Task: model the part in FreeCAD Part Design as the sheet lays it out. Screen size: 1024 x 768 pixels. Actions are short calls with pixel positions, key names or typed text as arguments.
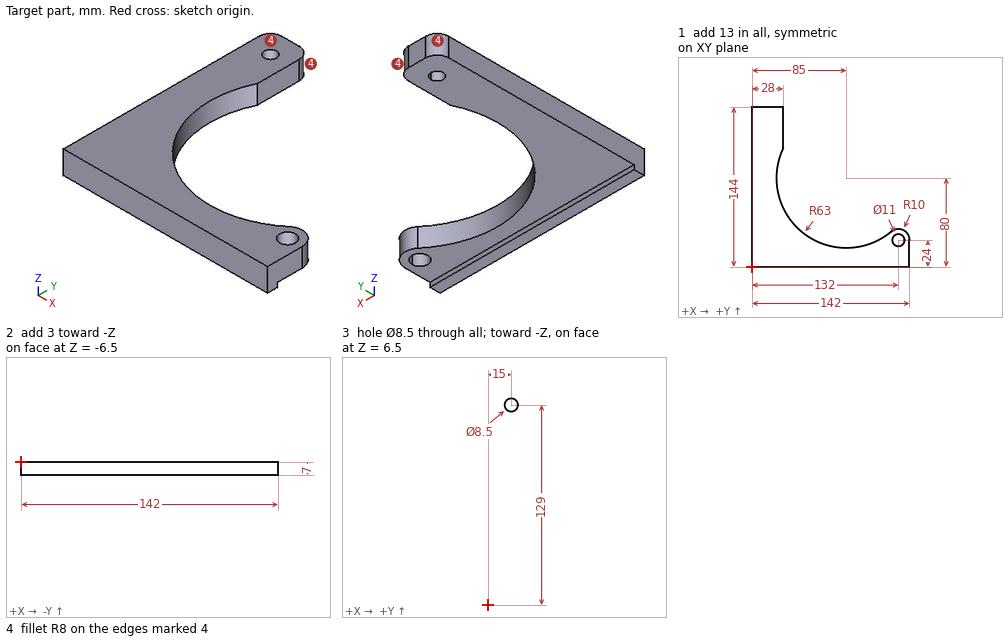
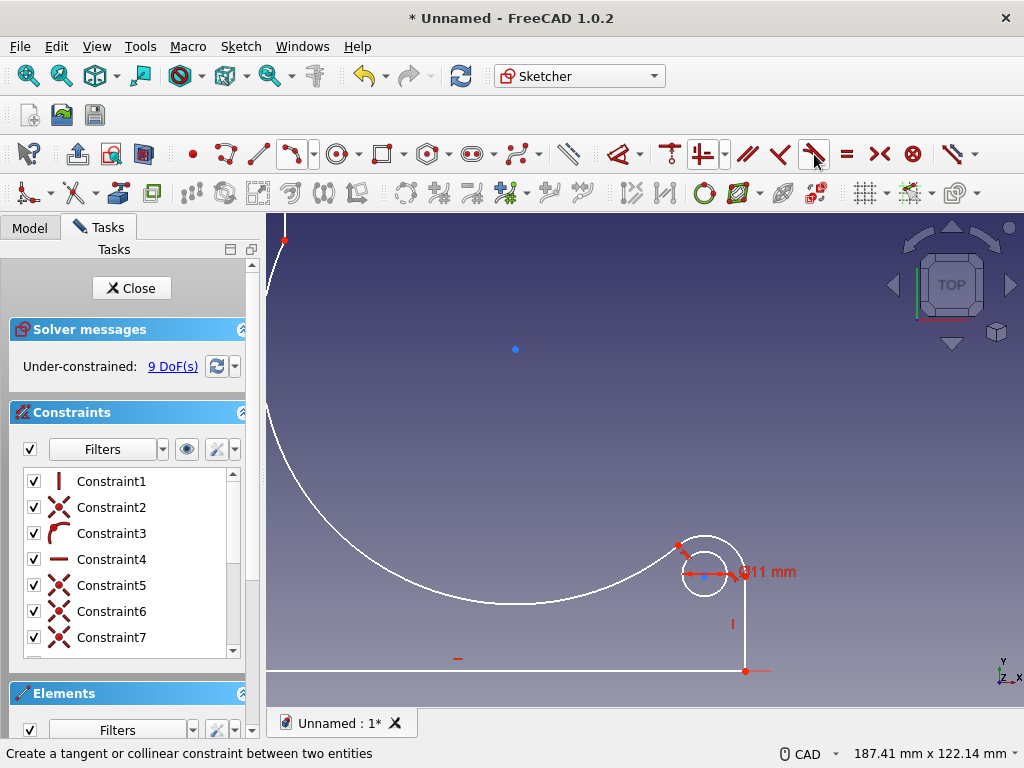
click(736, 551)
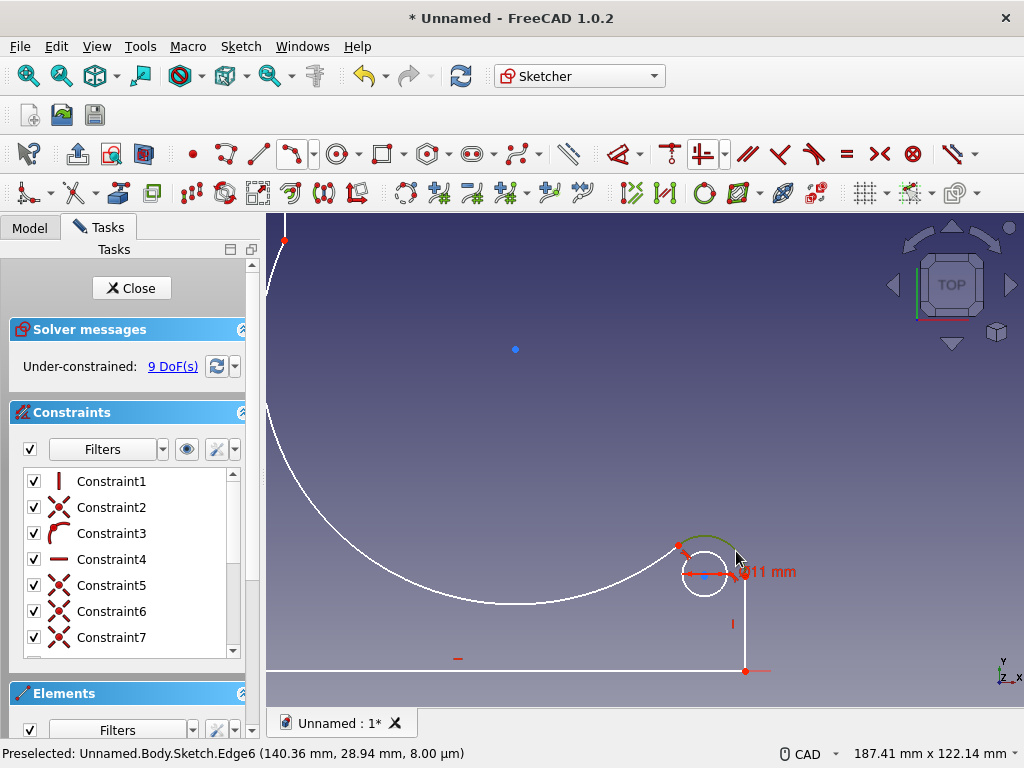
key(k)
key(r)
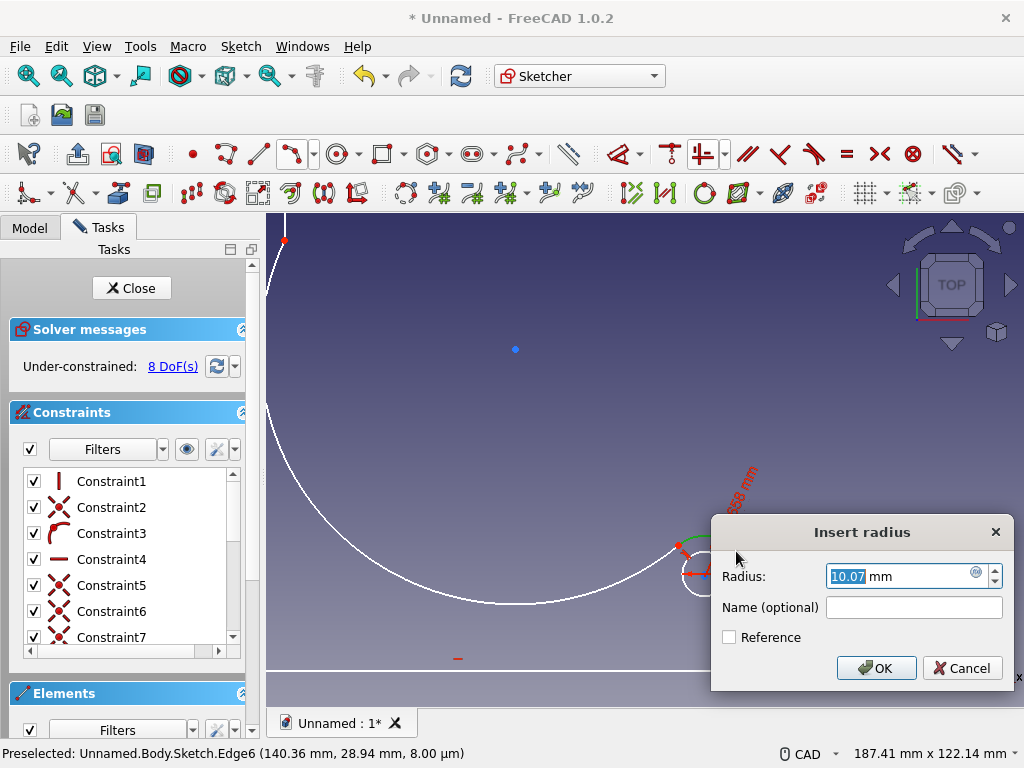
text(10)
key(Return)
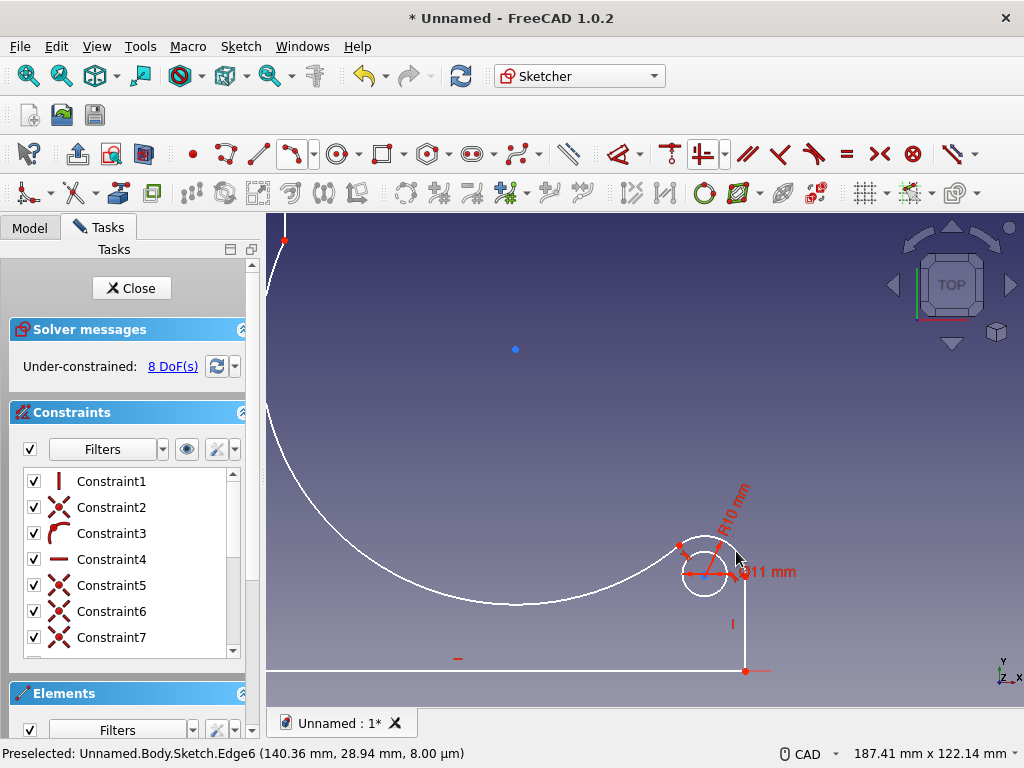
click(486, 603)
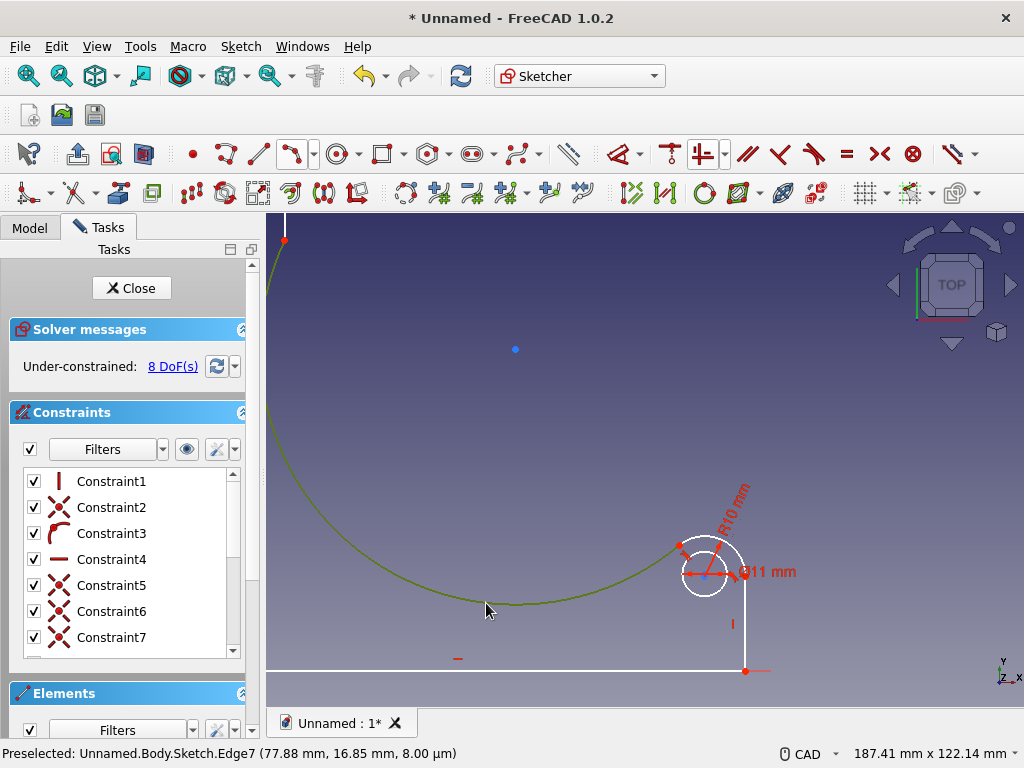
click(640, 154)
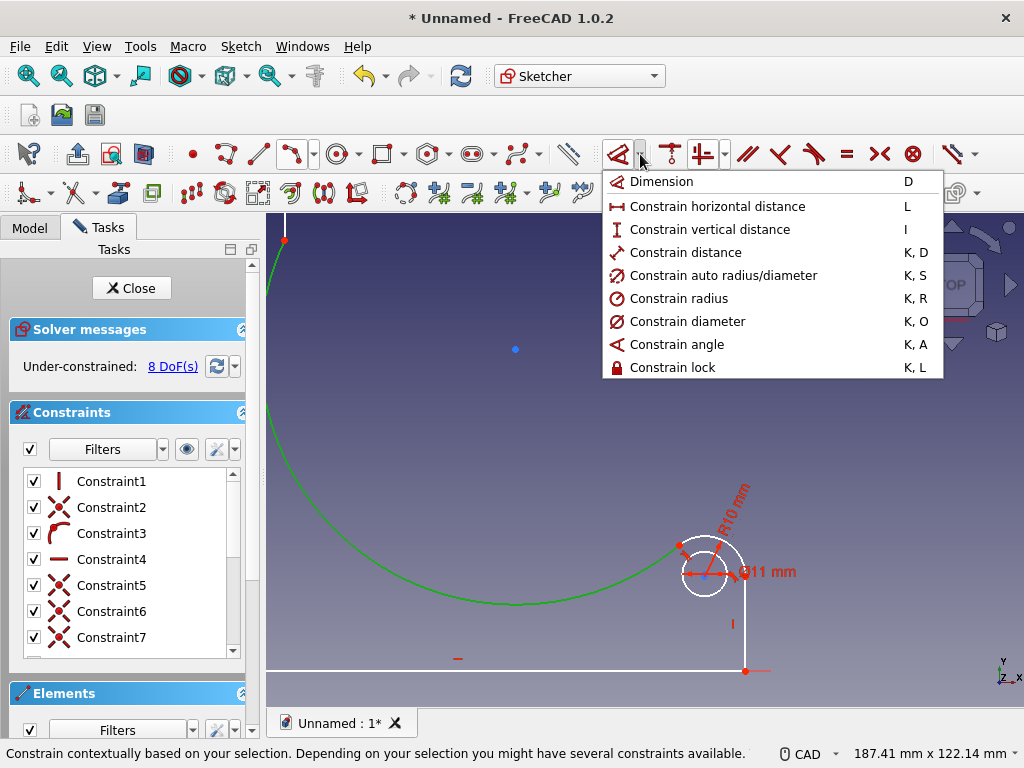
click(773, 298)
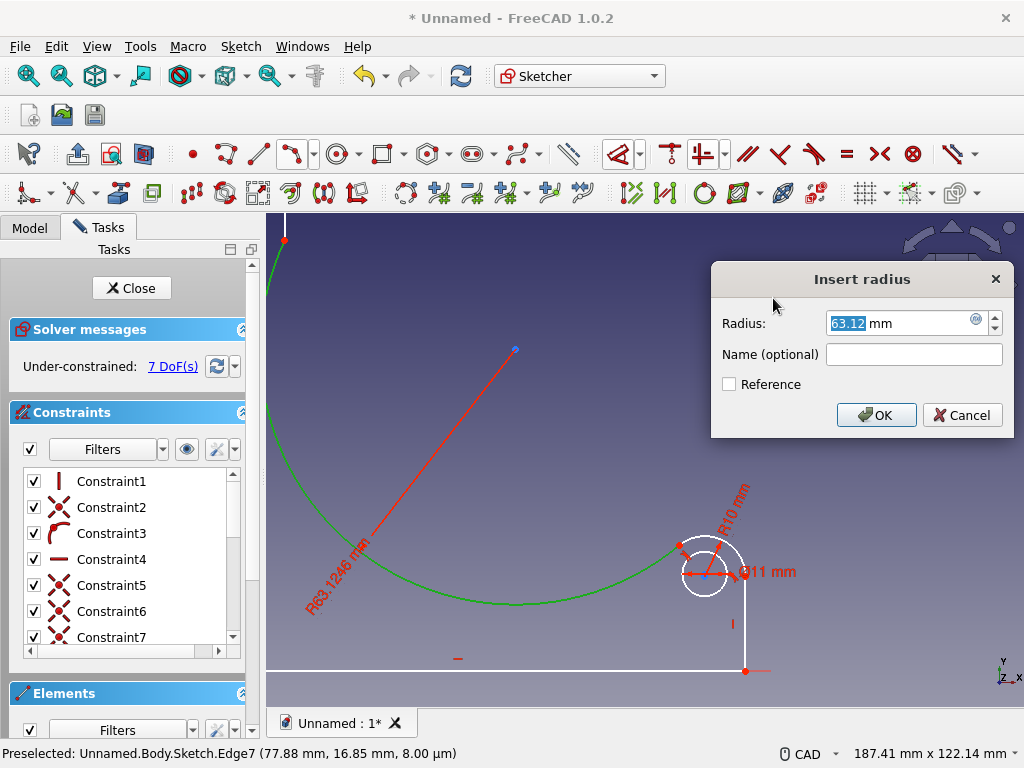
text(63)
key(Return)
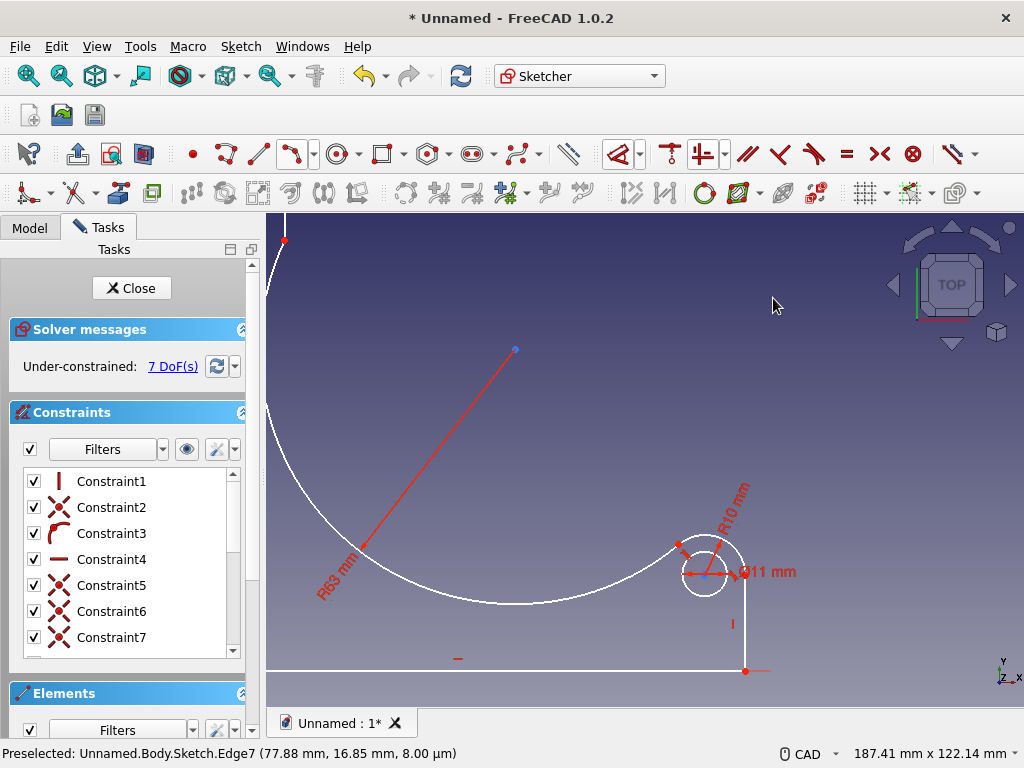
scroll(721, 557, down, 3)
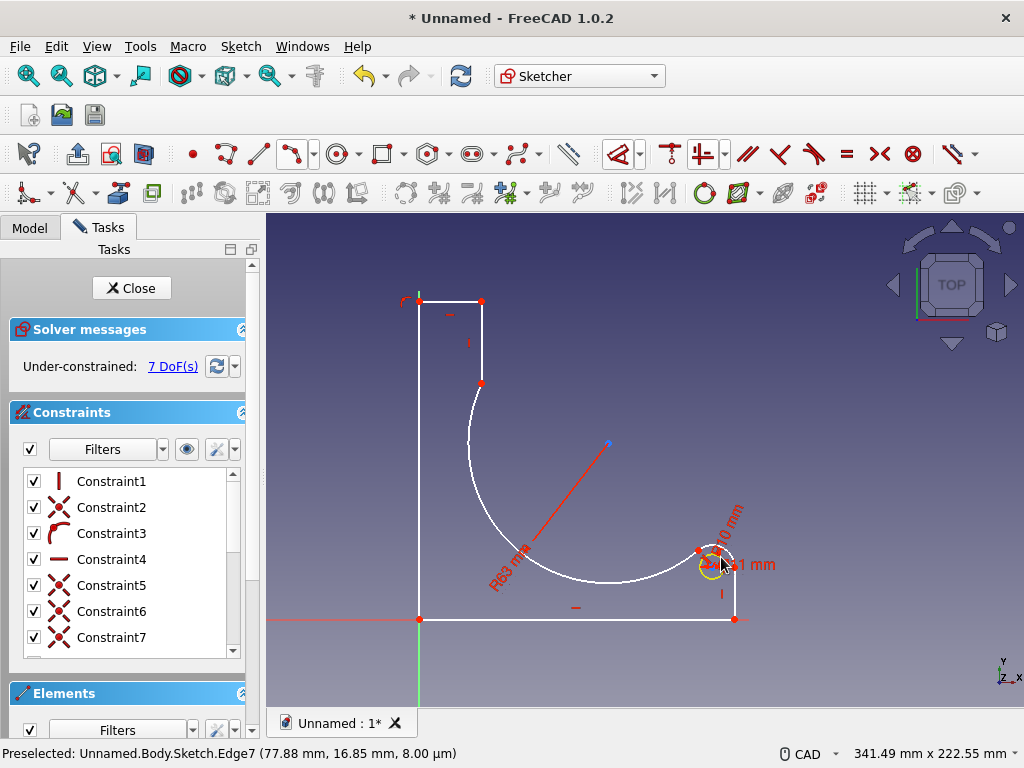
click(463, 302)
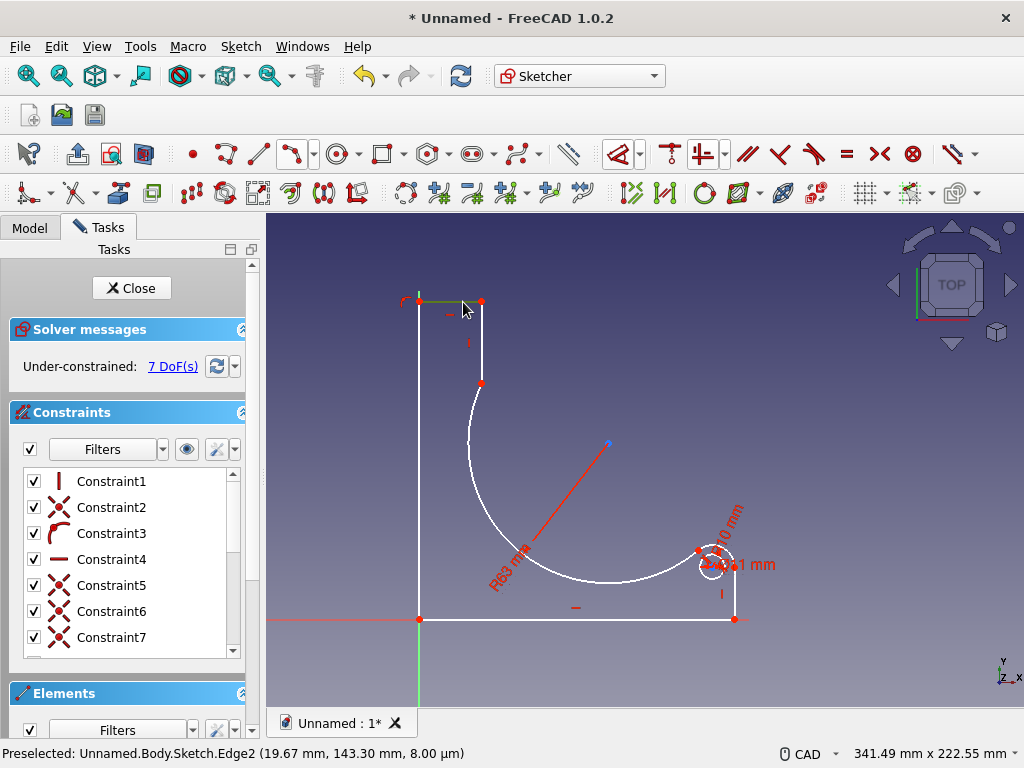
click(640, 154)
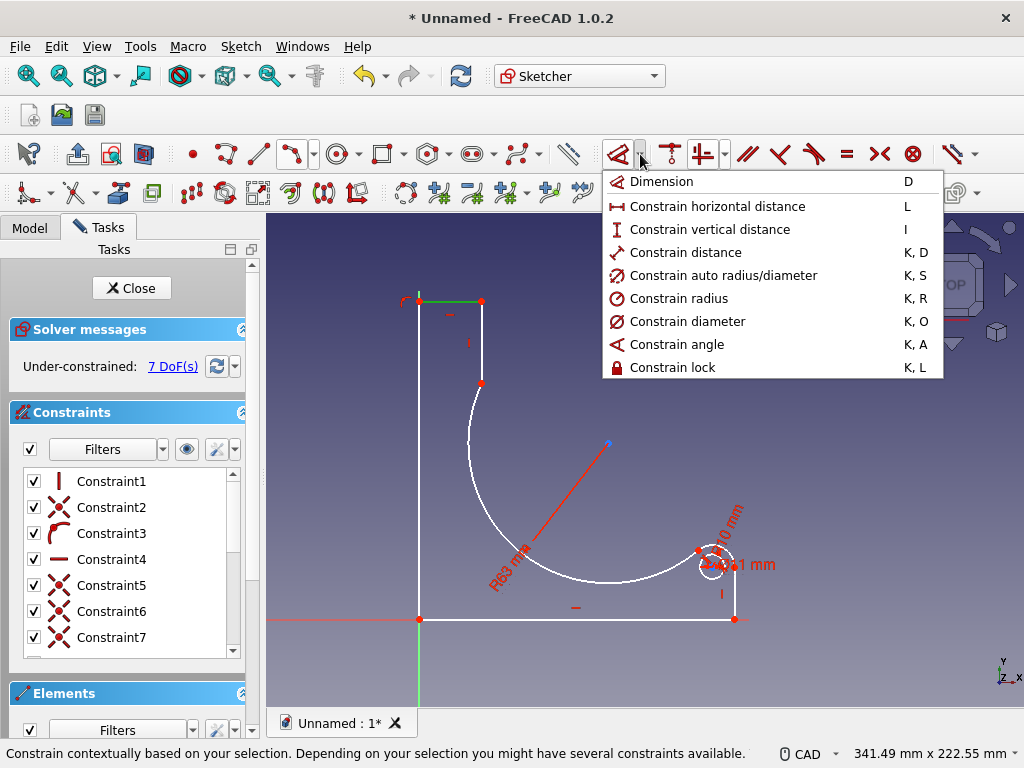
click(773, 206)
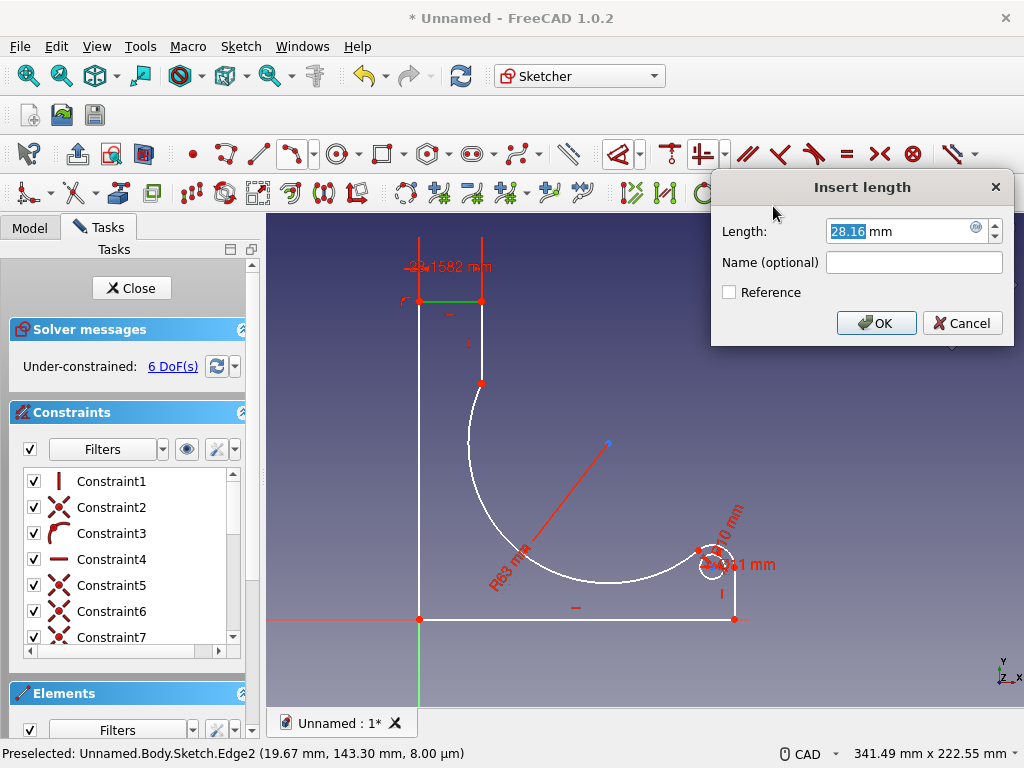
text(28)
key(Return)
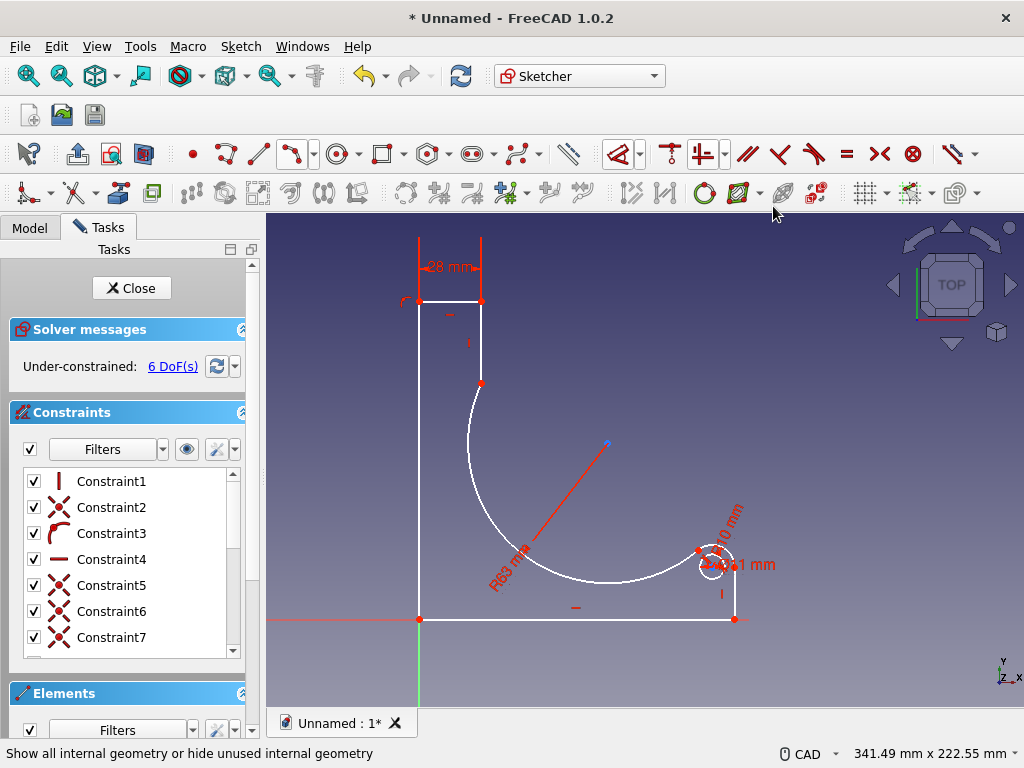
scroll(712, 567, up, 13)